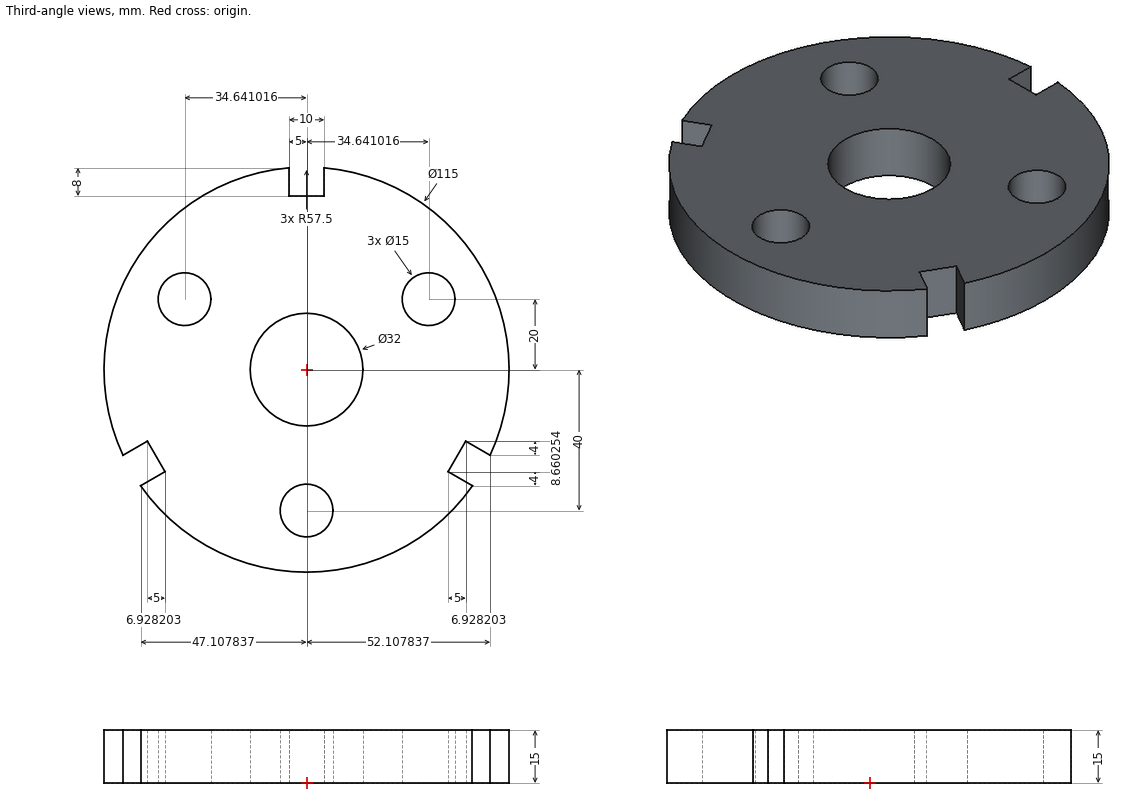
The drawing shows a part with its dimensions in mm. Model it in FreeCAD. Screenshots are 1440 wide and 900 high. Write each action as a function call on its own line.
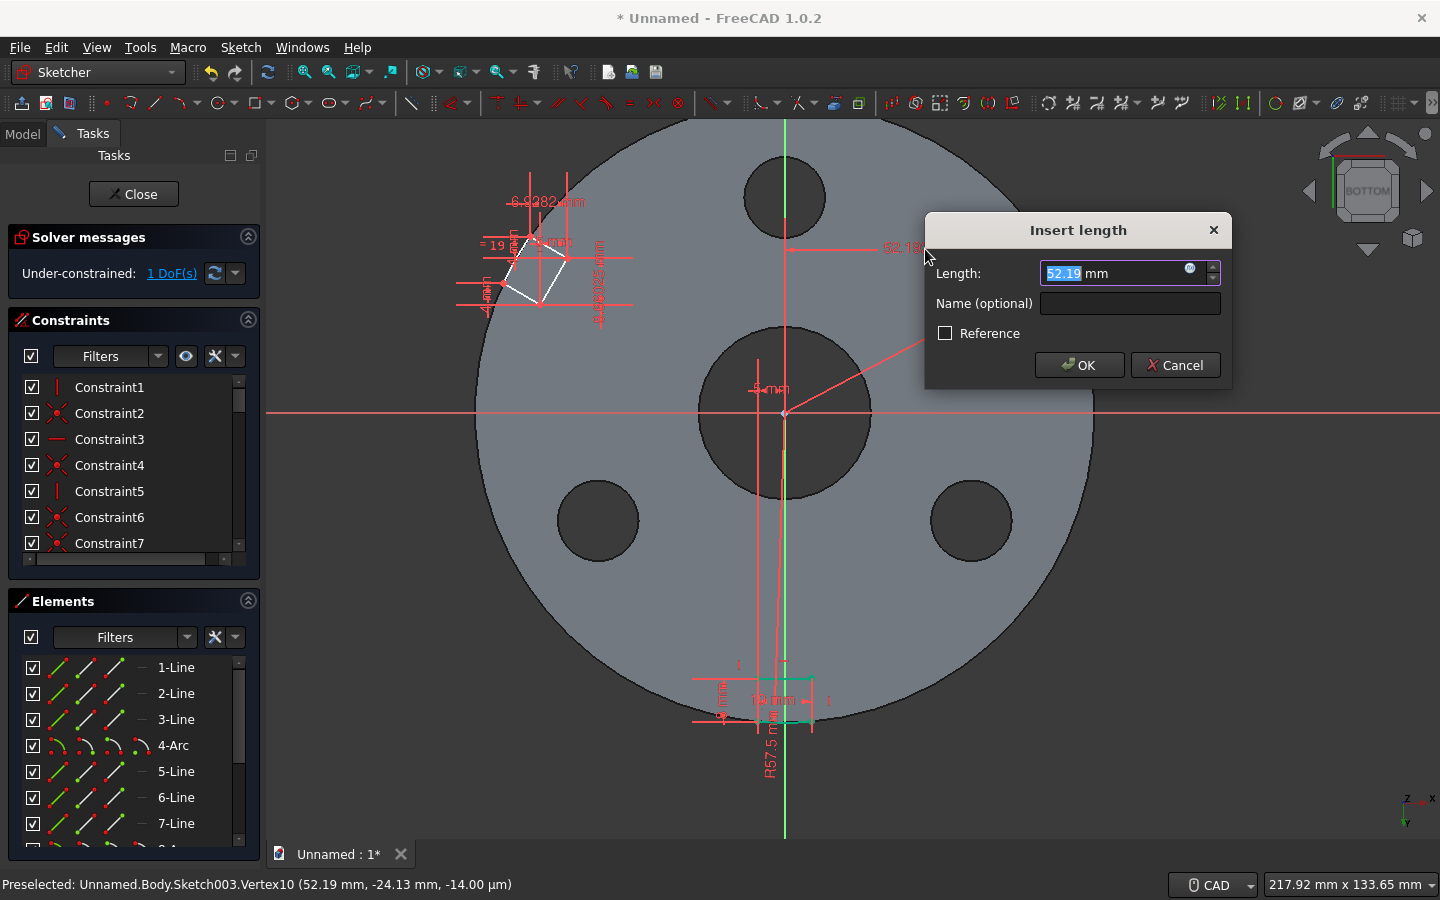
text(52.107837)
key(Return)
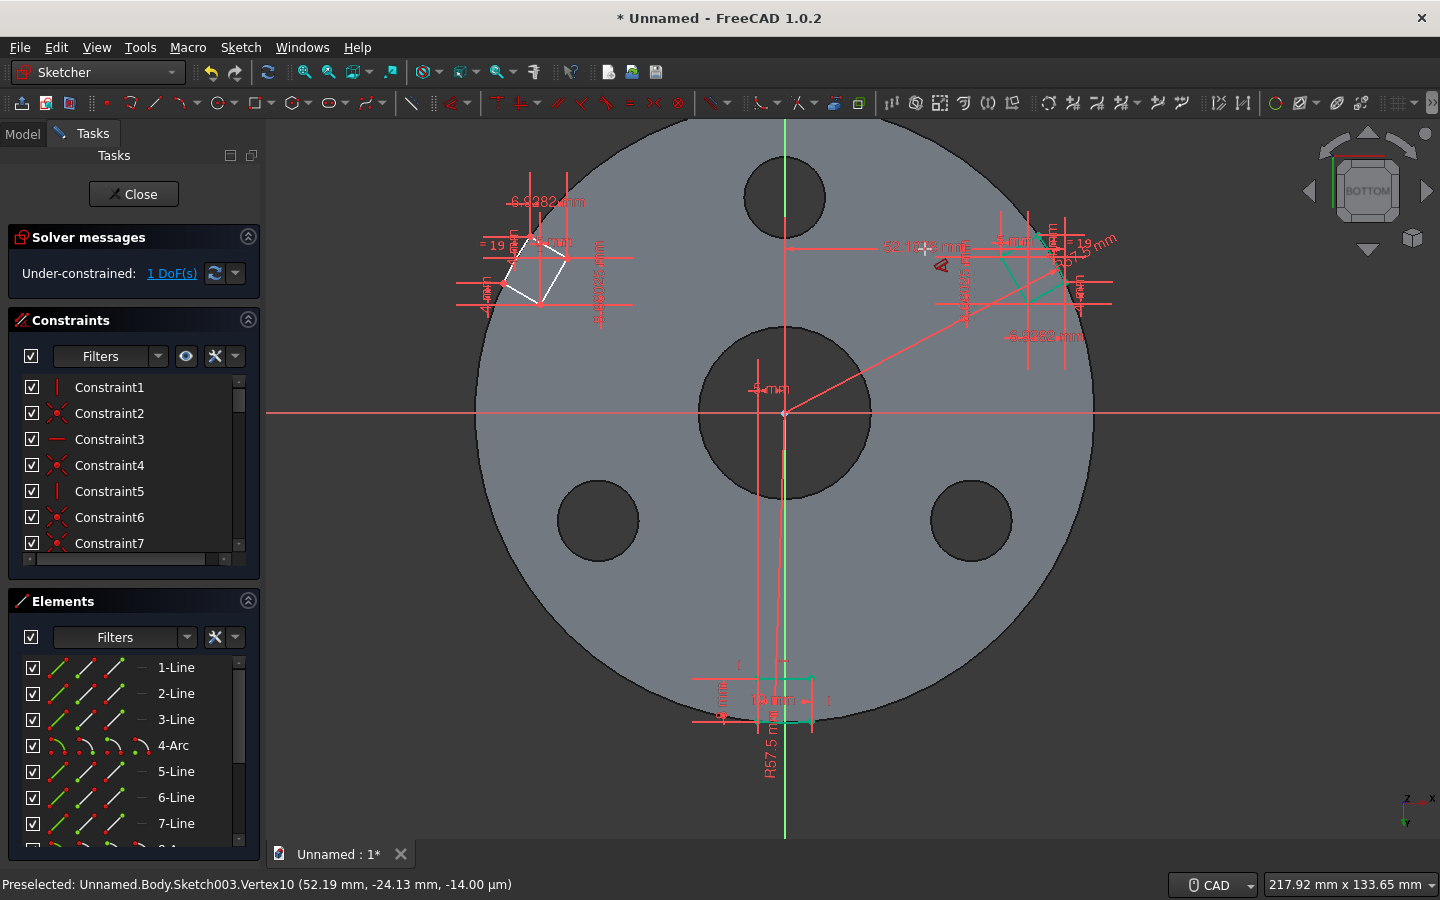
click(530, 237)
click(657, 203)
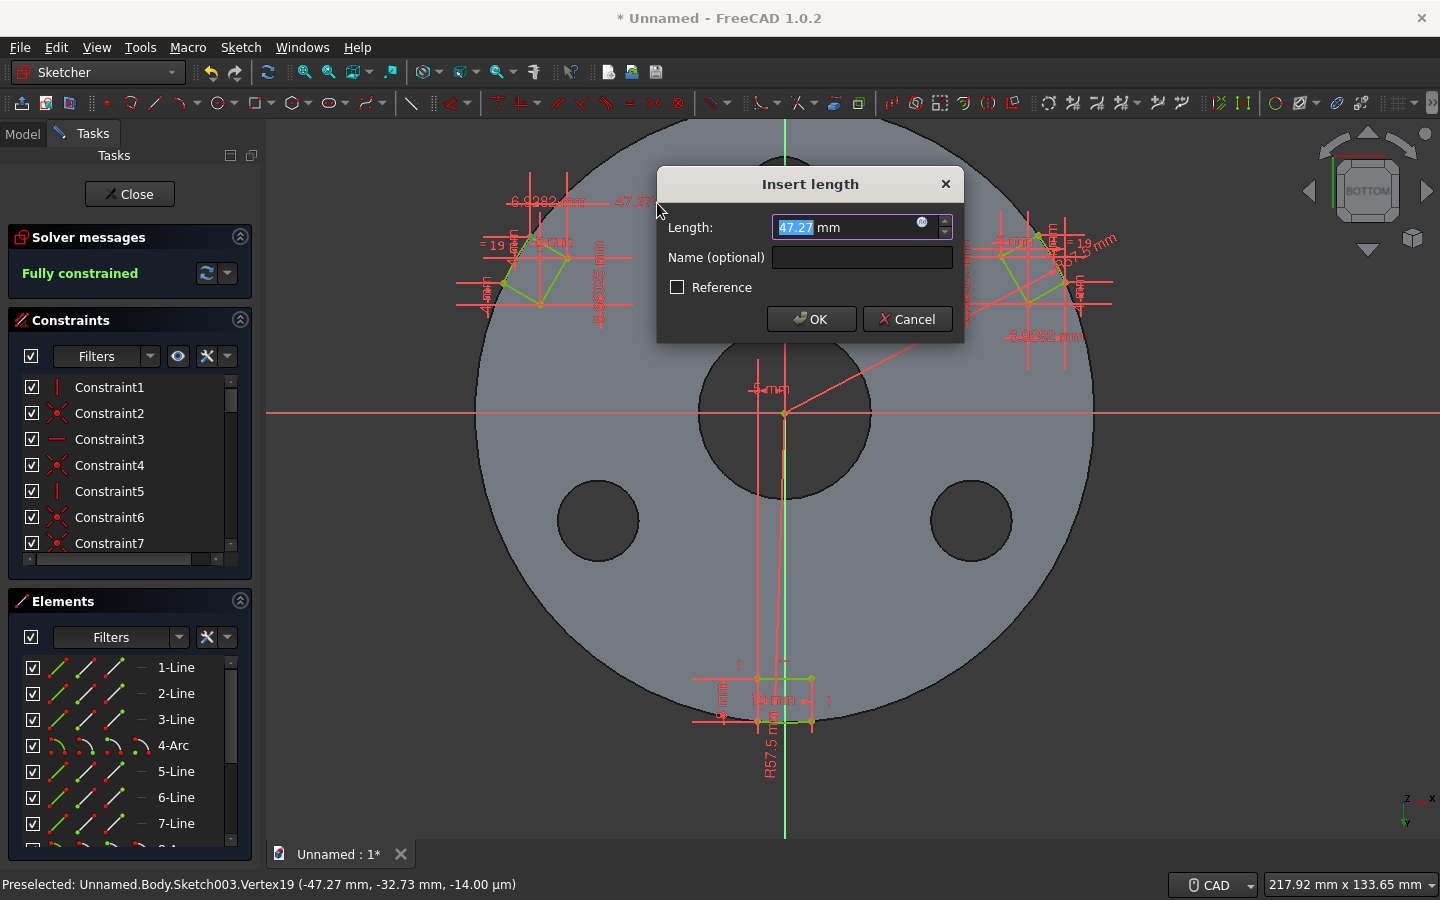
text(47.107837)
key(Return)
key(Escape)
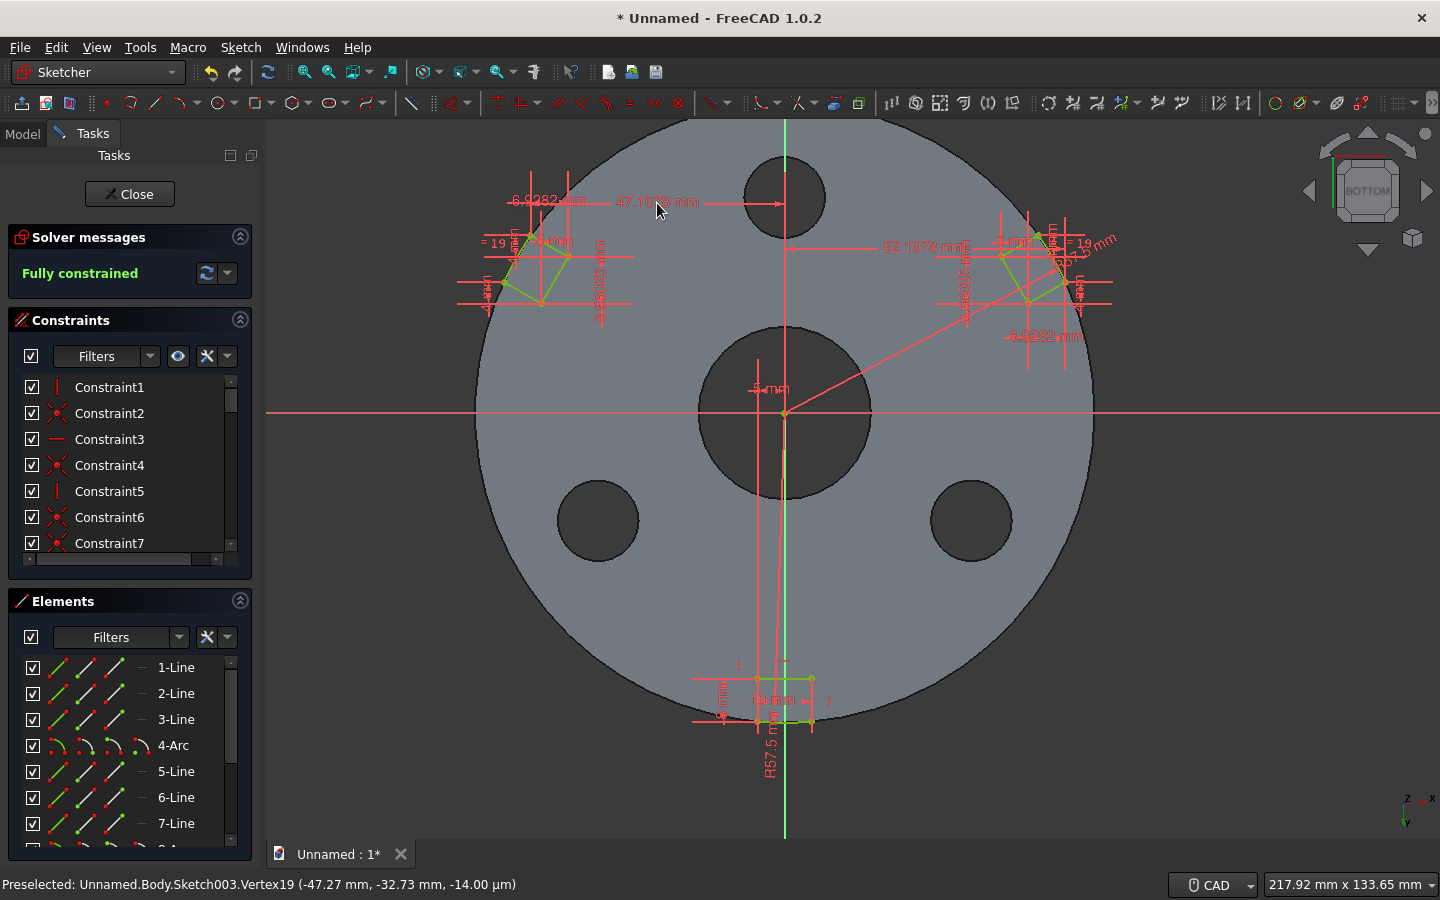
click(130, 194)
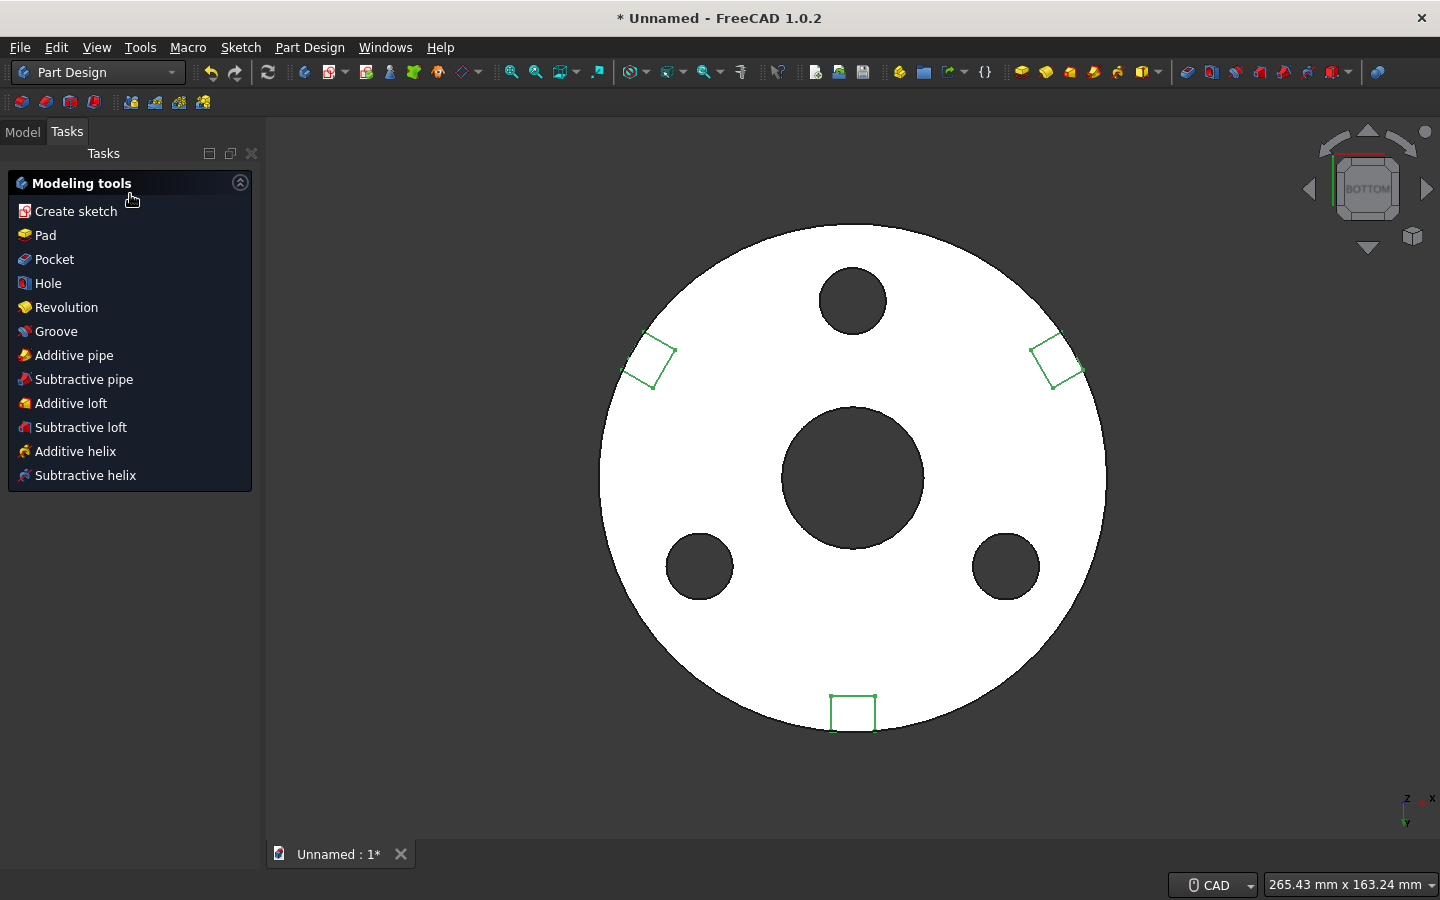
click(1188, 72)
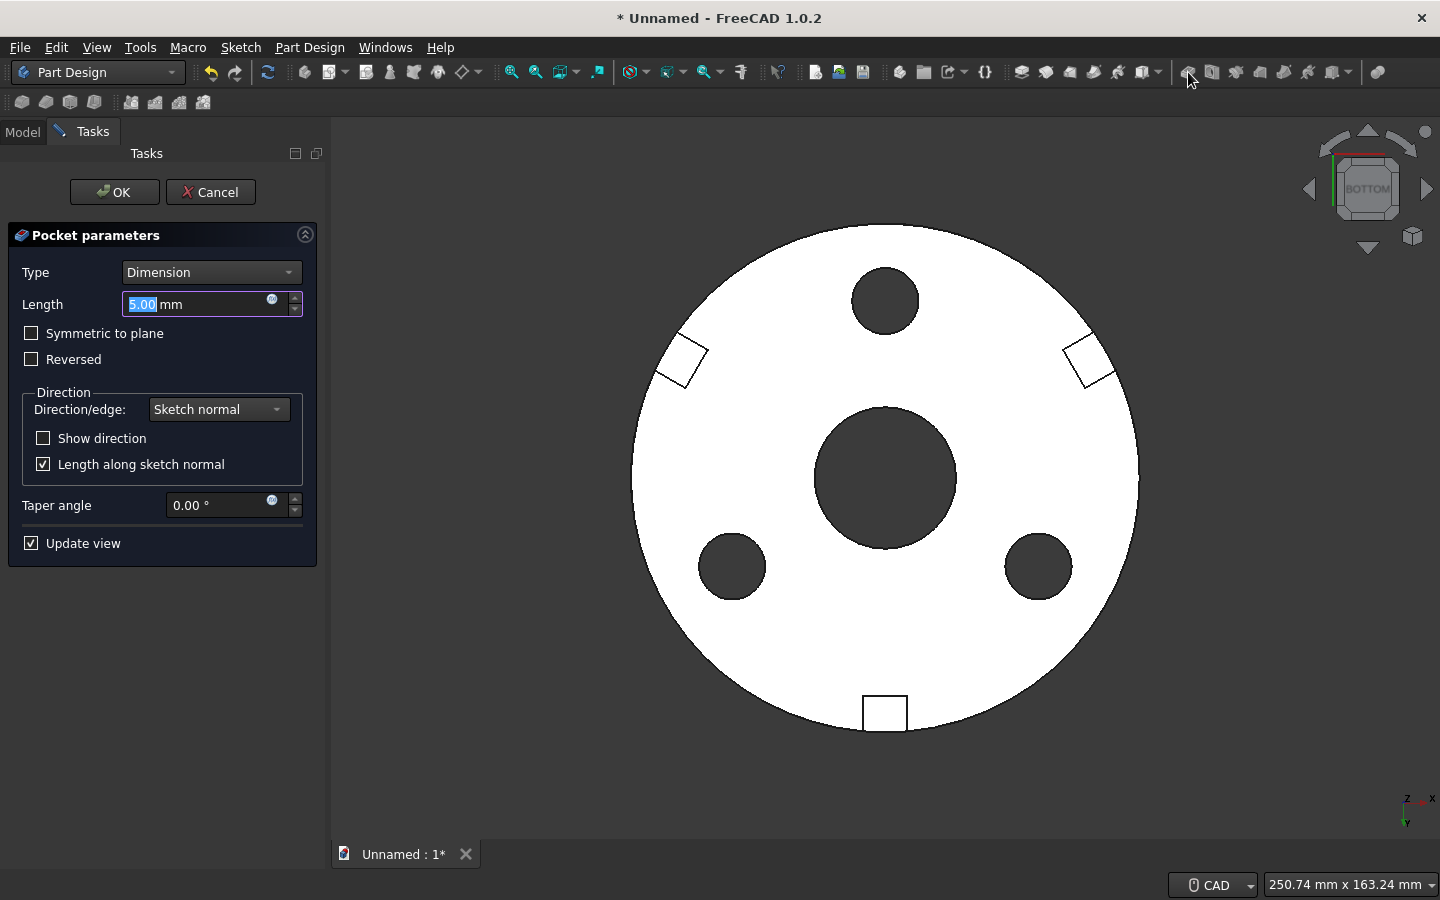
text(15)
key(Tab)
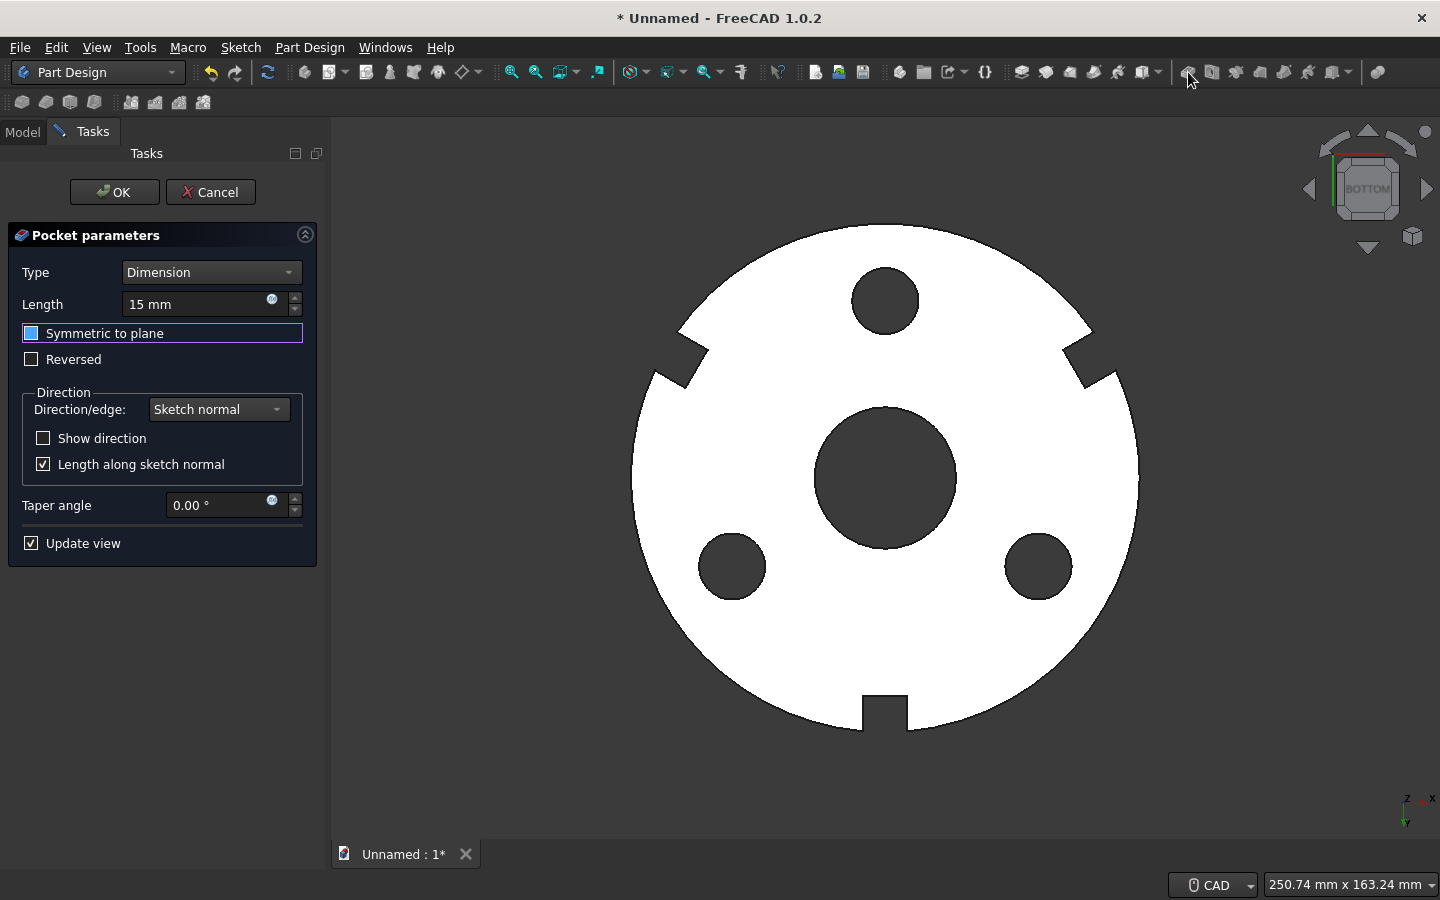
click(115, 192)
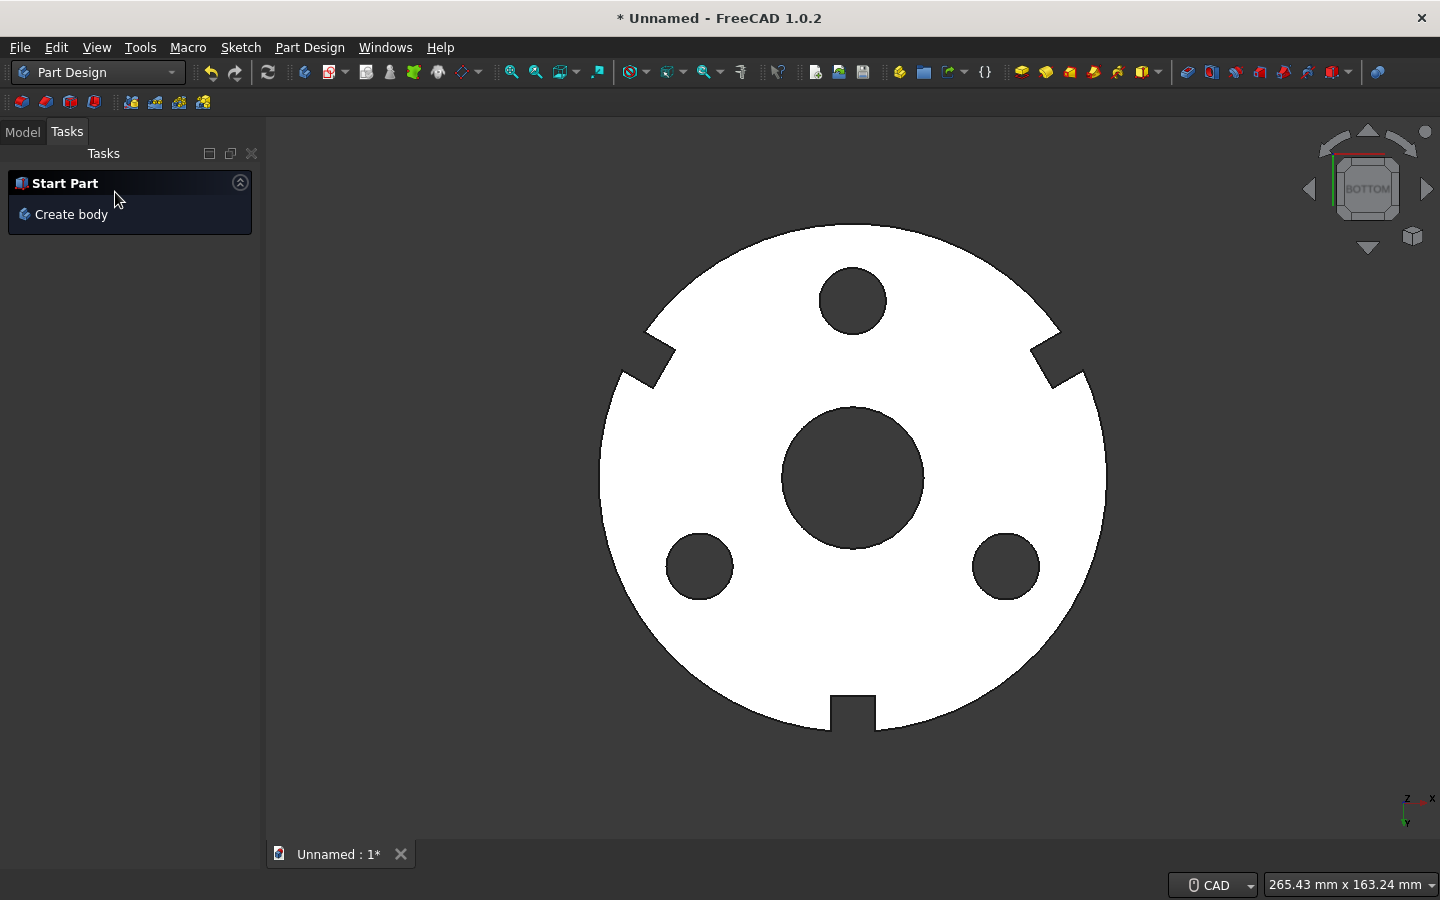
key(0)